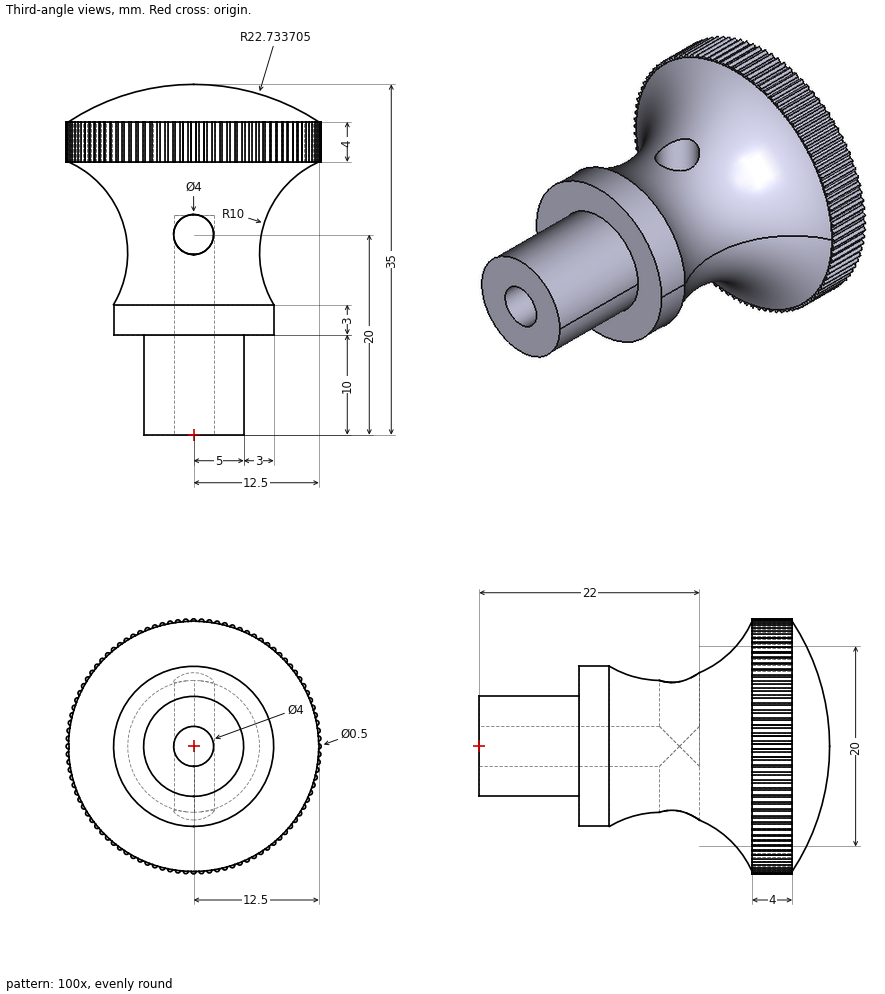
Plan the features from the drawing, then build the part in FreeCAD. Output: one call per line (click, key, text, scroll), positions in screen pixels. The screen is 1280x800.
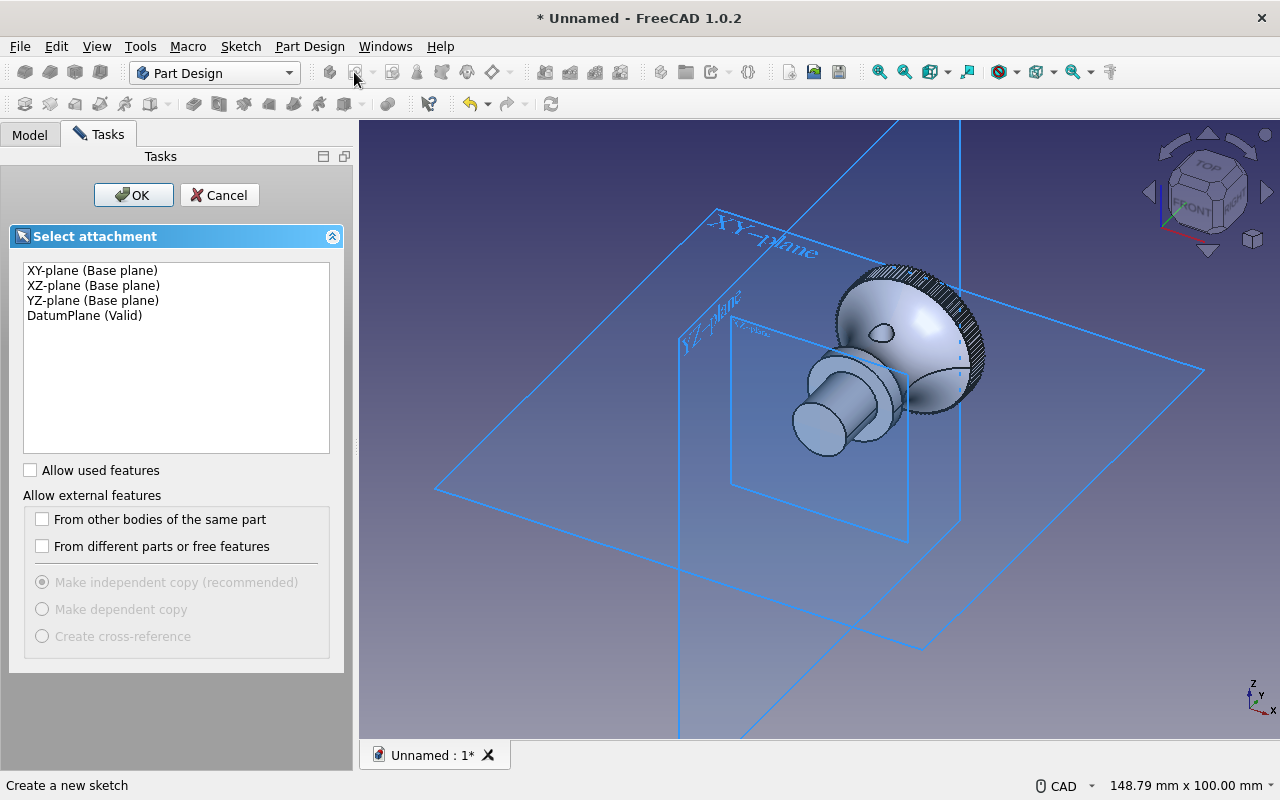
click(84, 286)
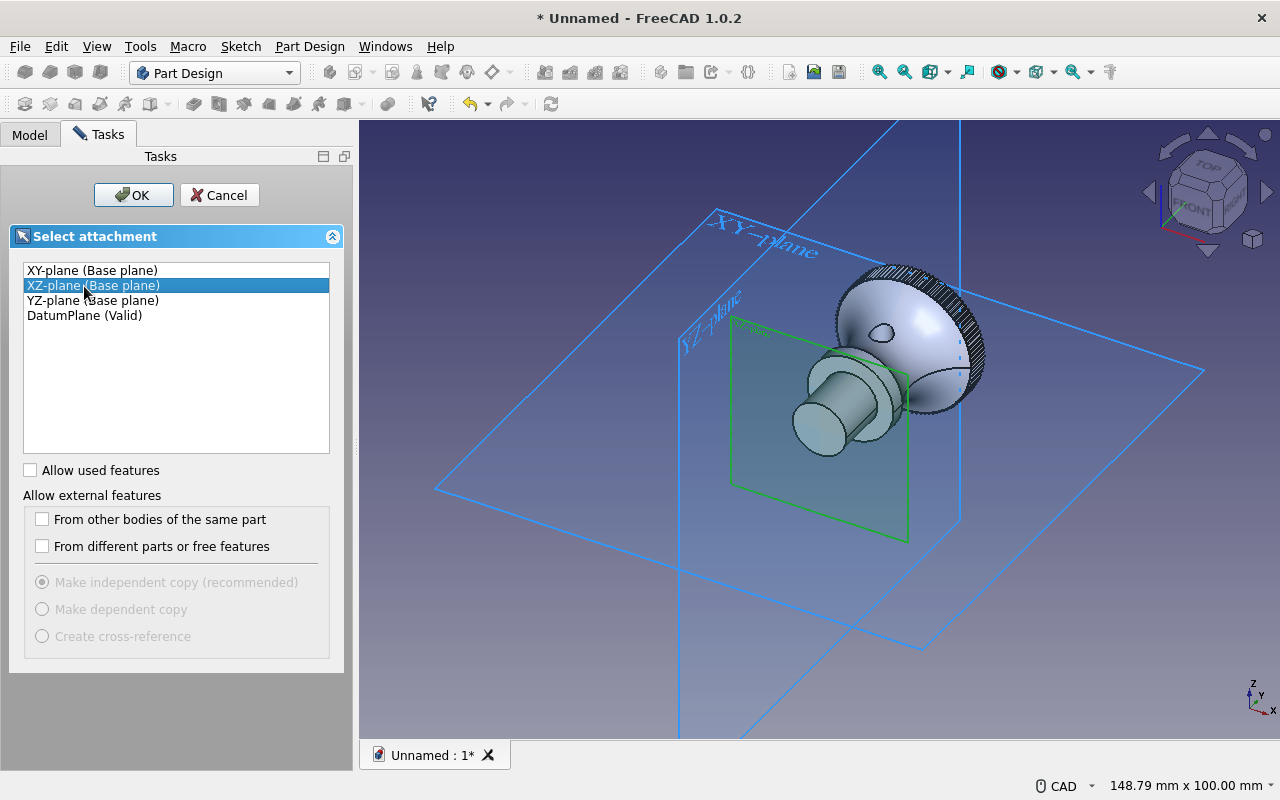
click(134, 195)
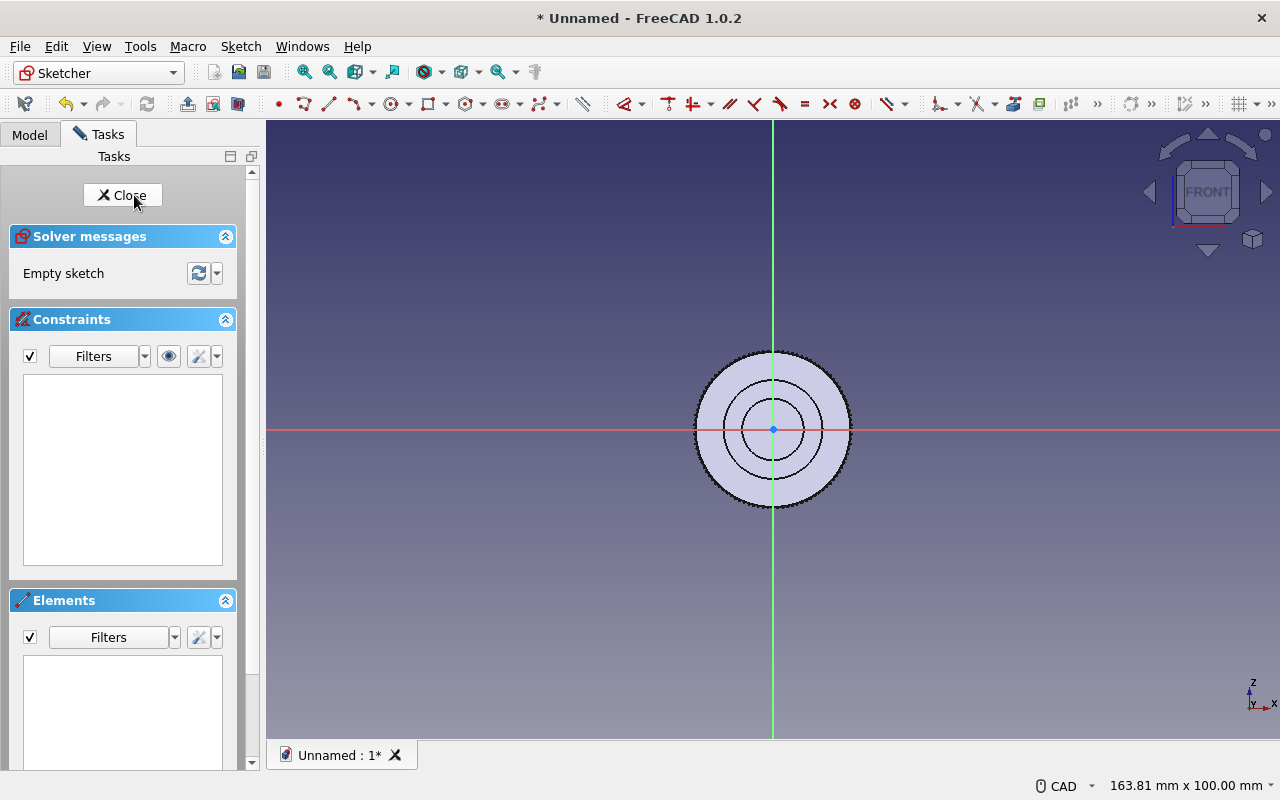
scroll(777, 430, up, 14)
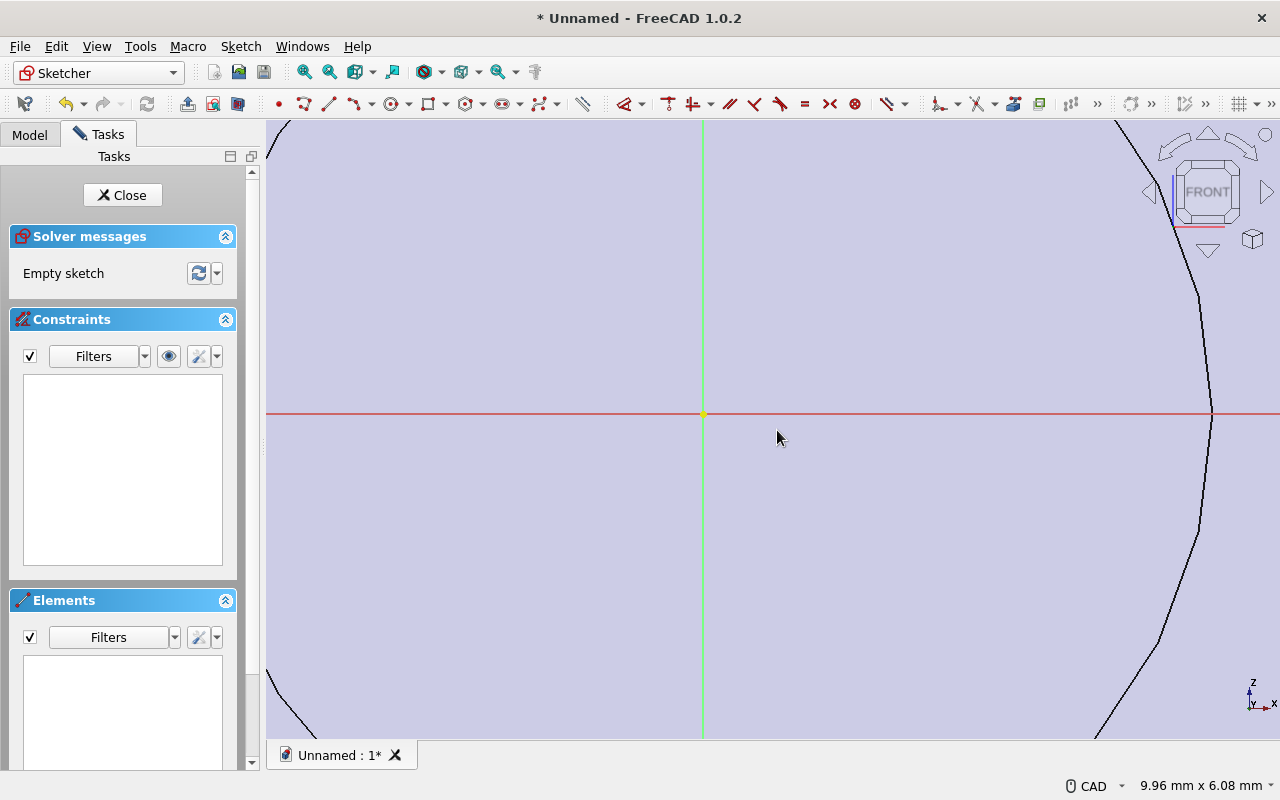
click(390, 104)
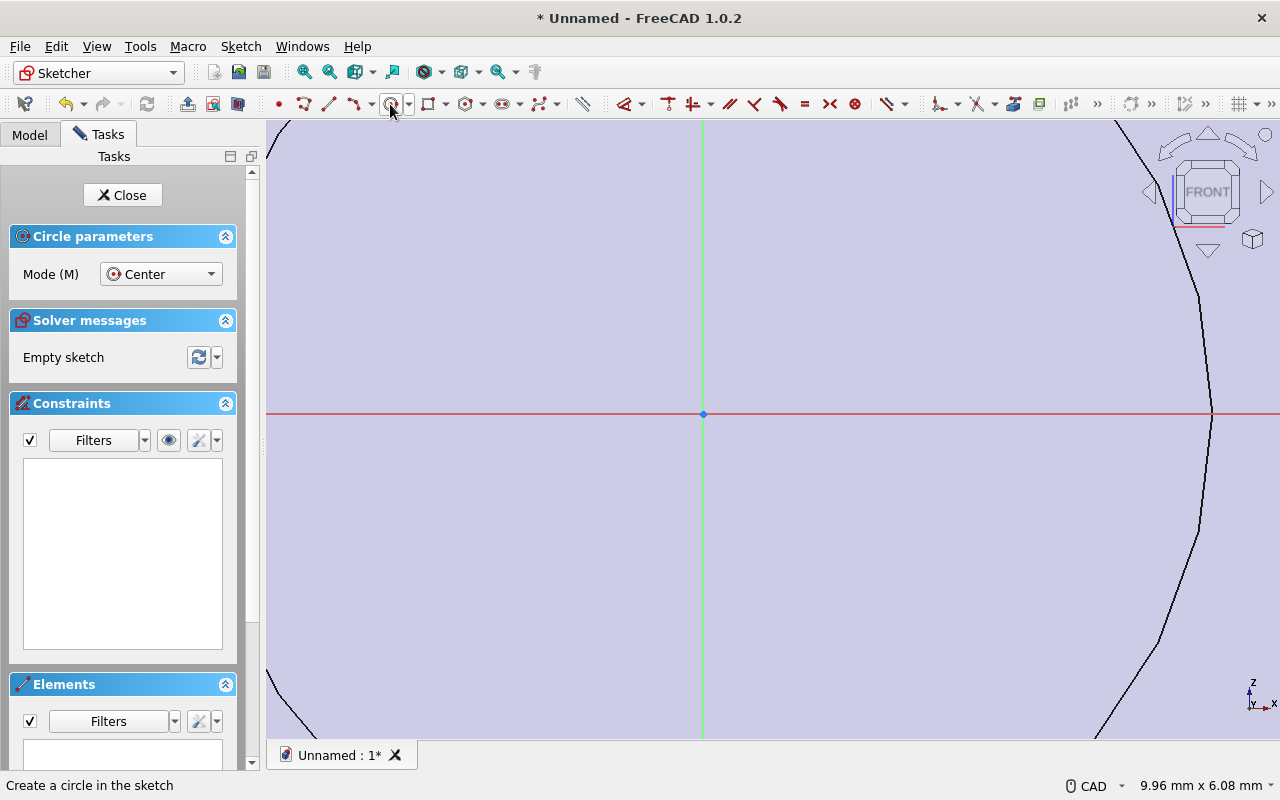
click(703, 414)
move(847, 270)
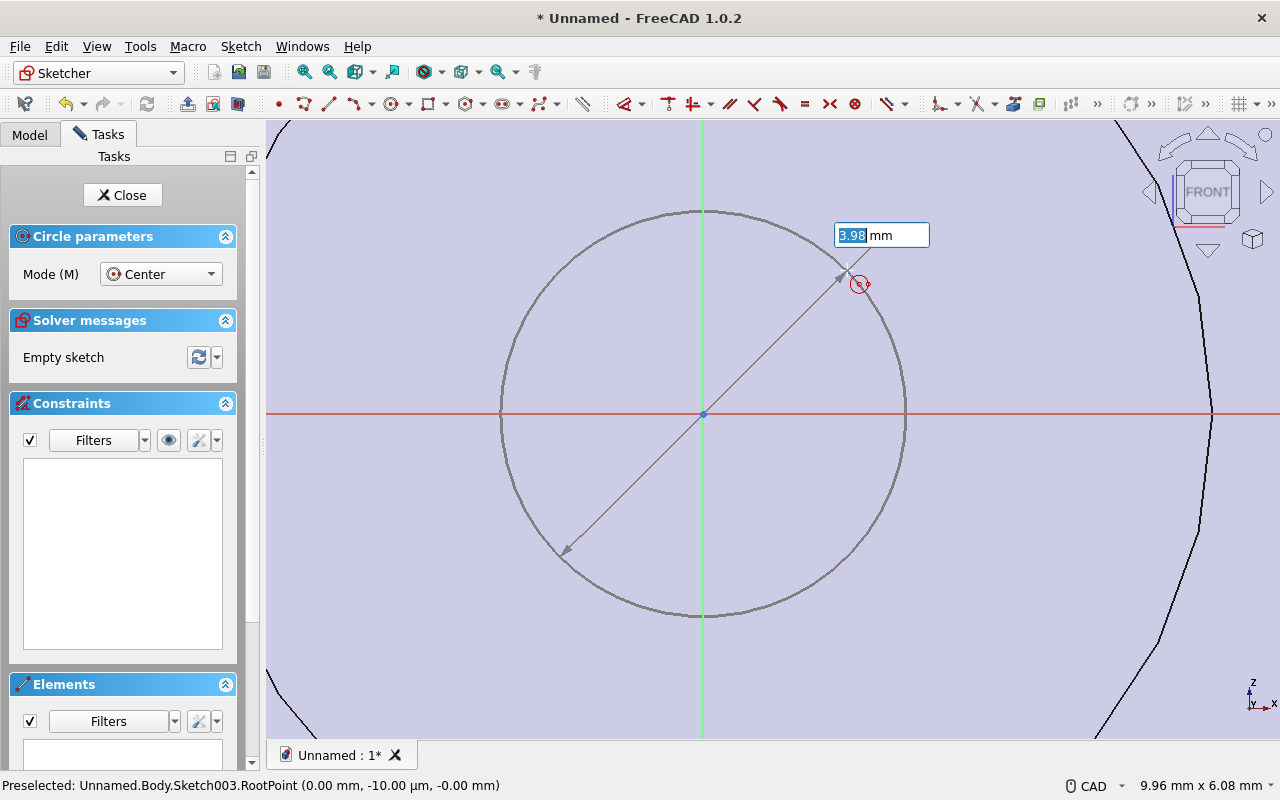
text(4)
key(Return)
key(Escape)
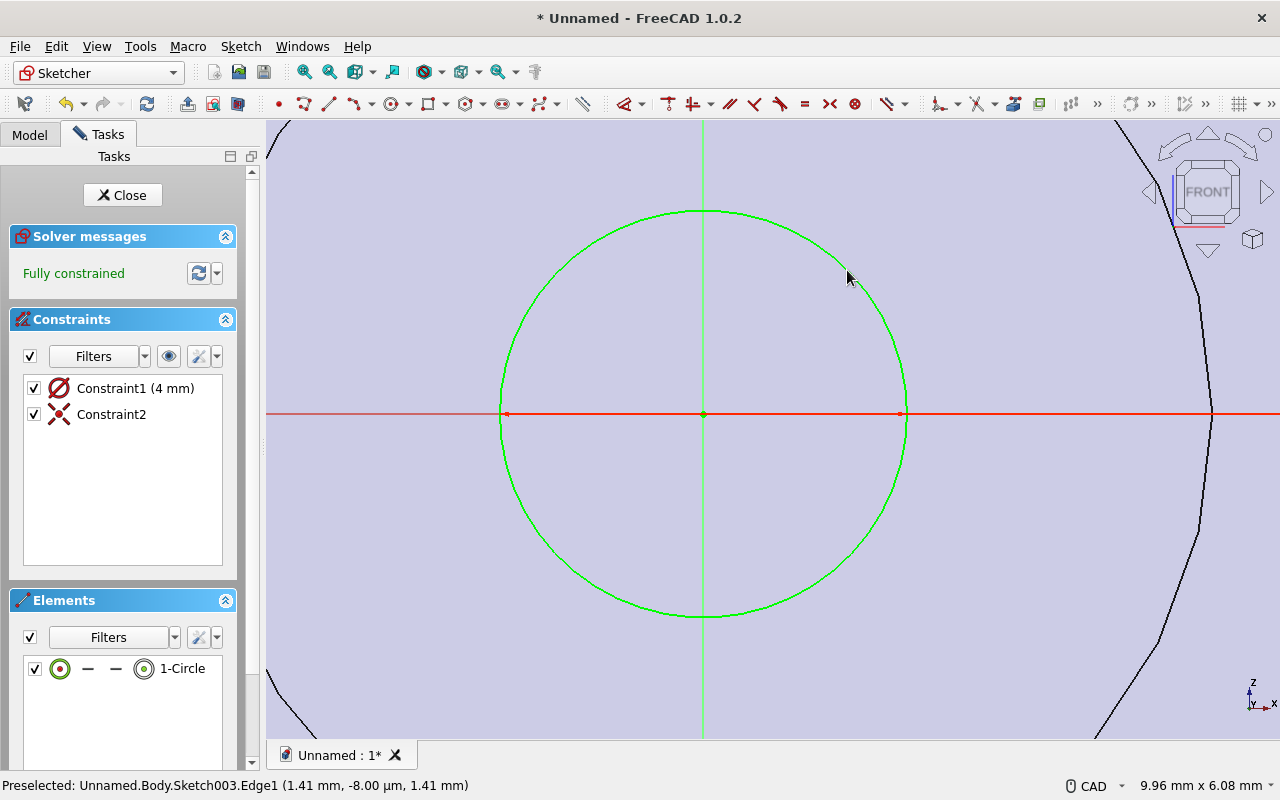
click(123, 195)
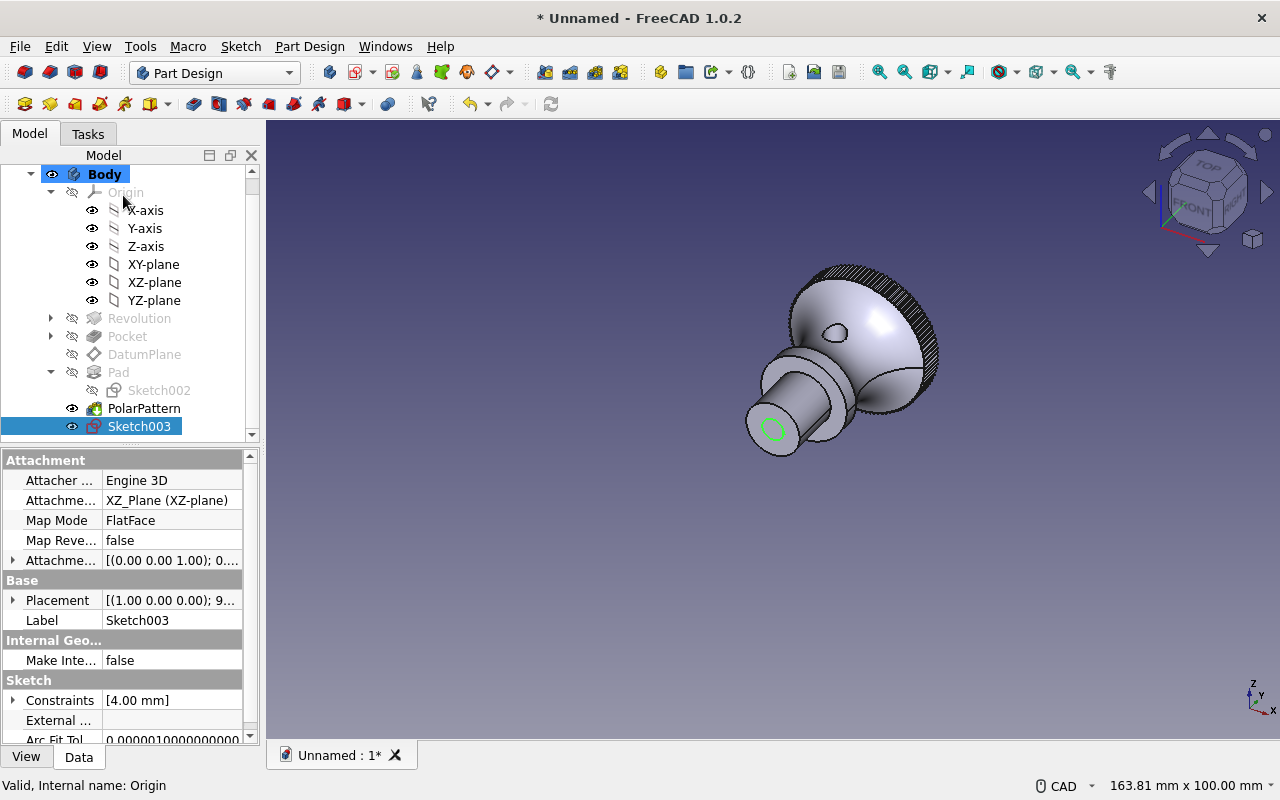
click(194, 104)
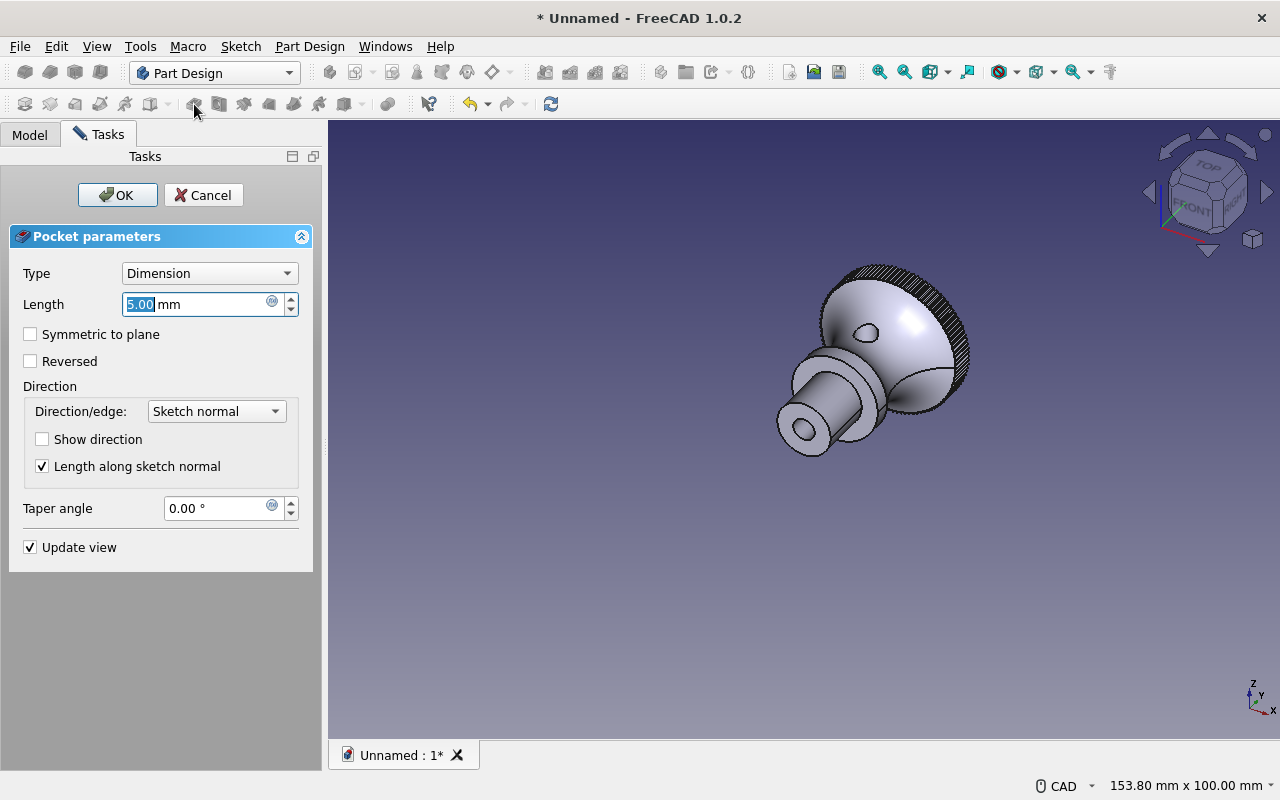
text(22)
key(Tab)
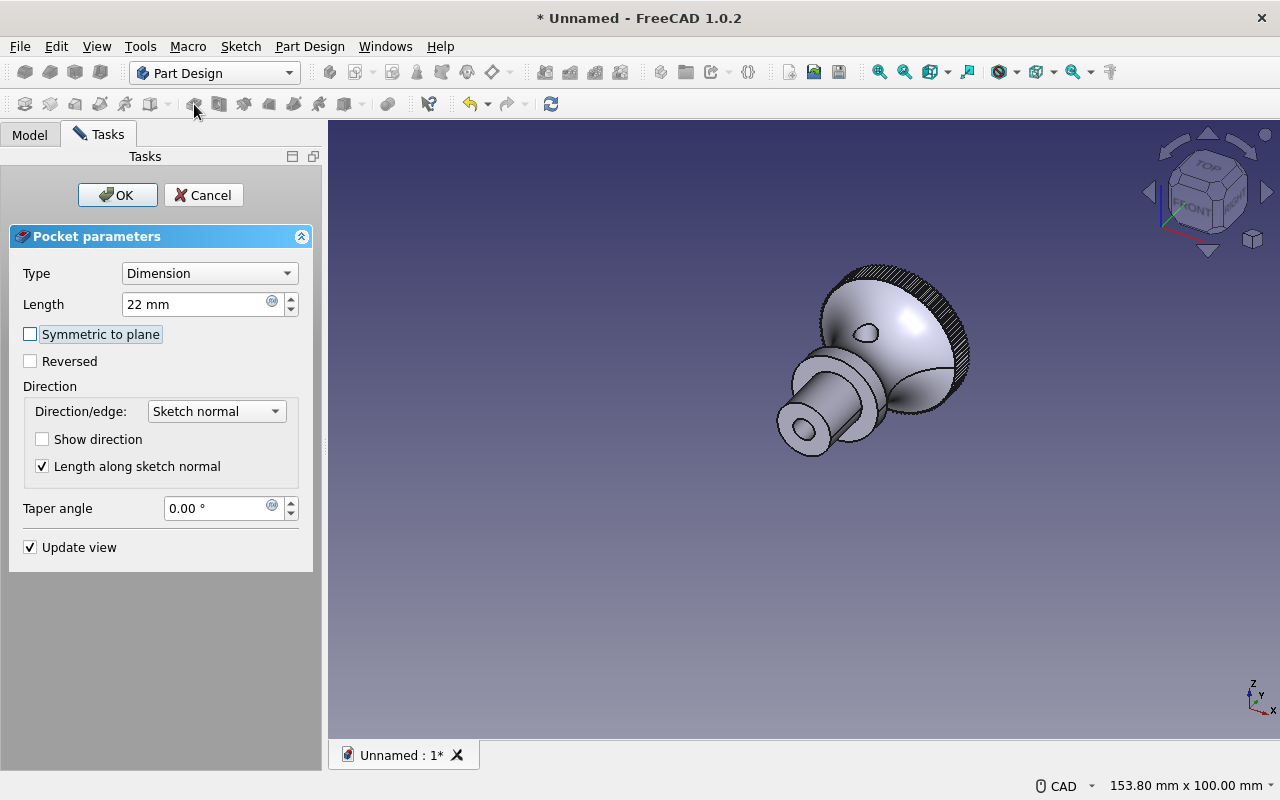
click(118, 195)